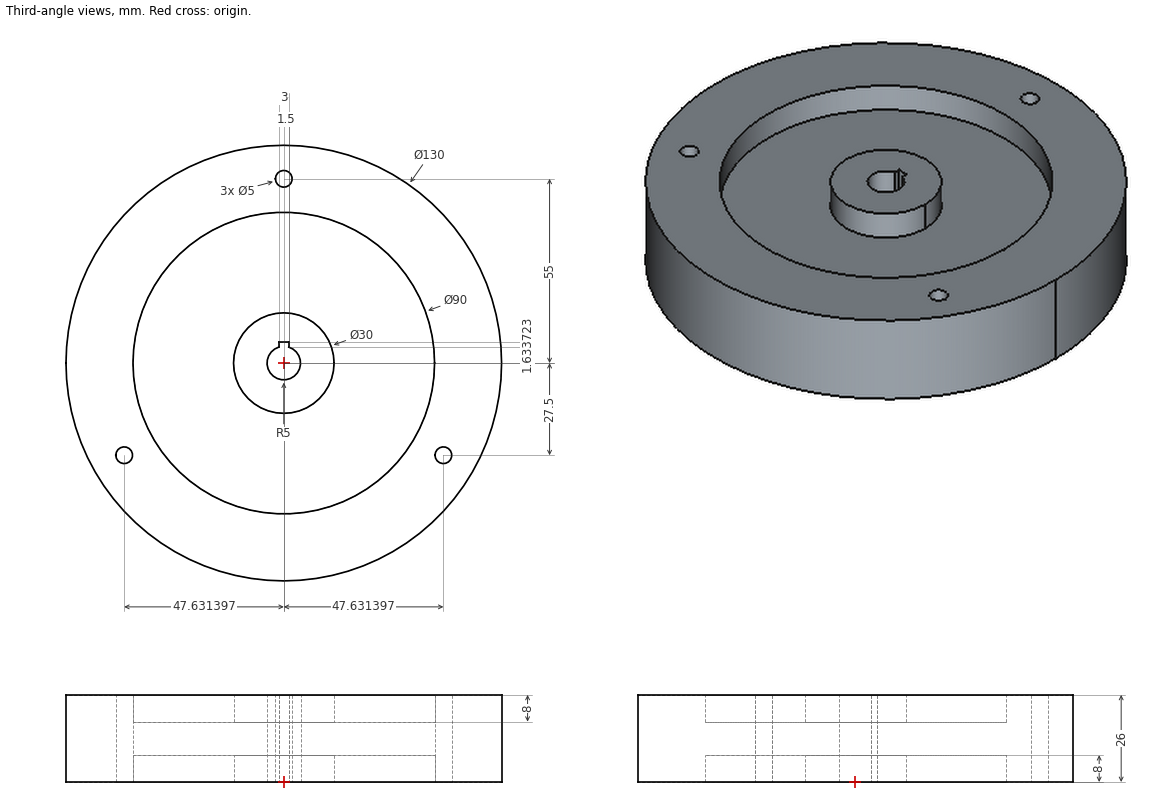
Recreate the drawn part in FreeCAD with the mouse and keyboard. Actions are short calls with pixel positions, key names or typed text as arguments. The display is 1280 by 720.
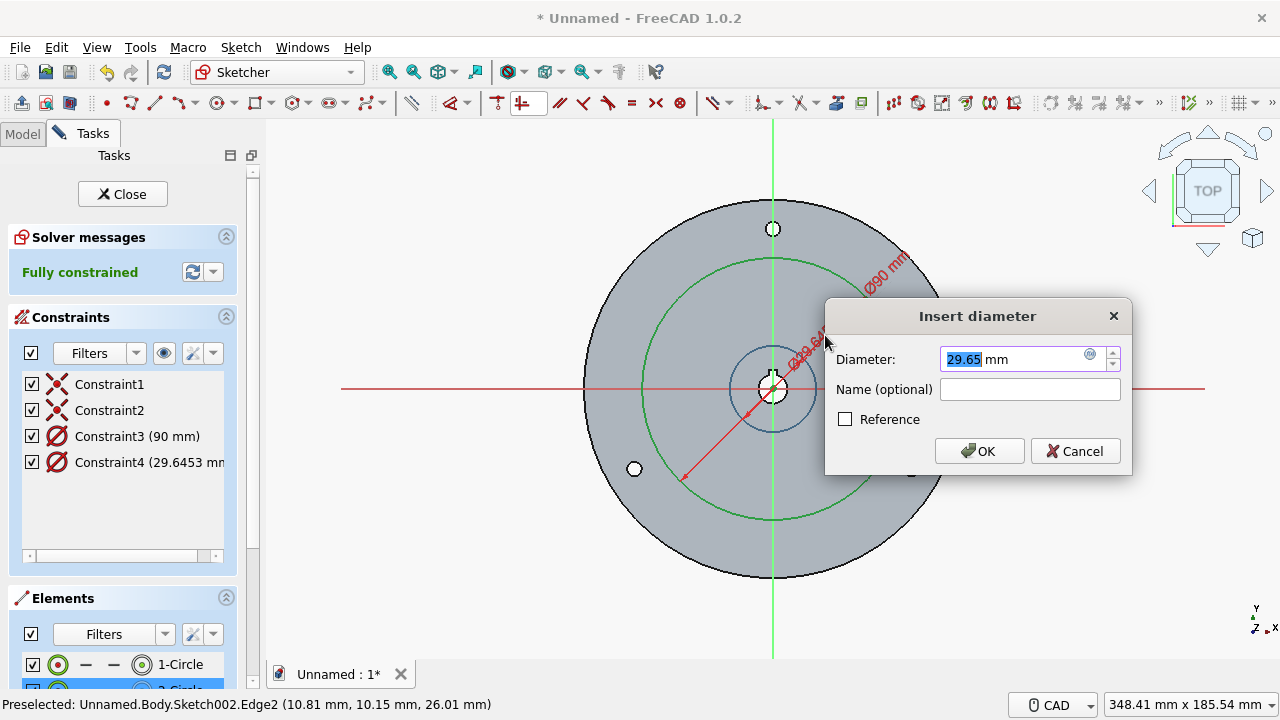
text(30)
key(Return)
key(Escape)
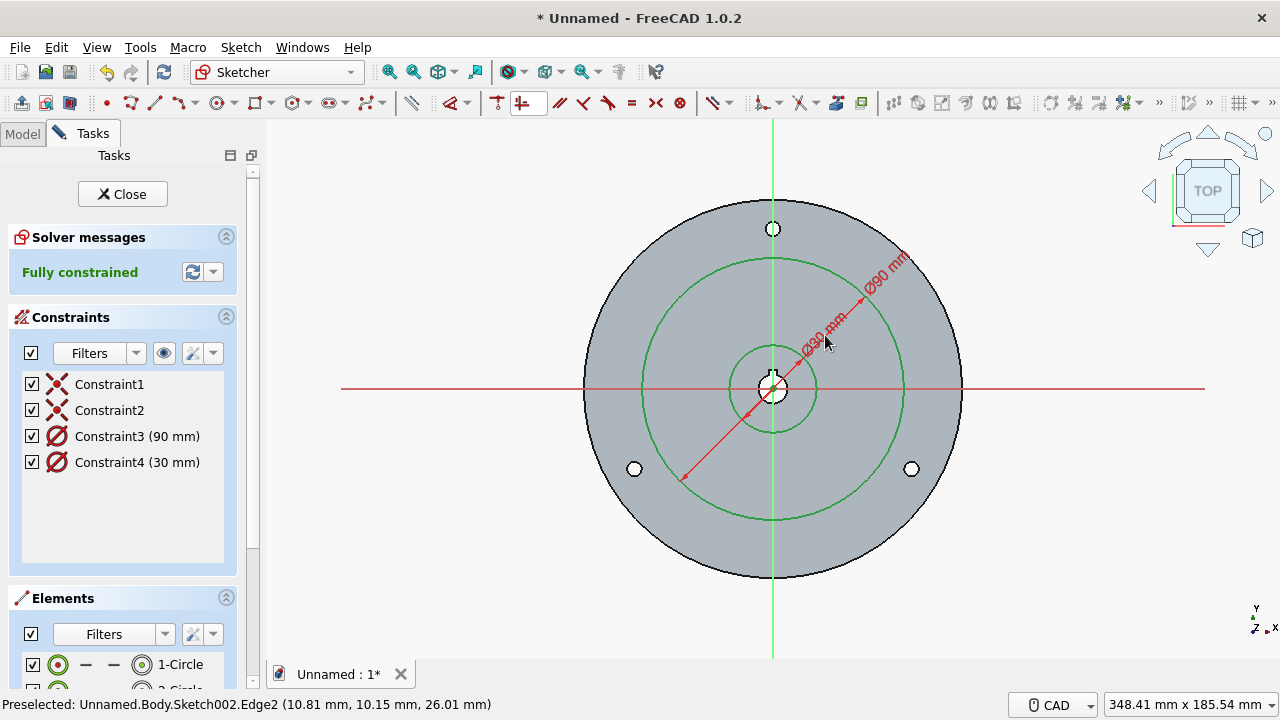
click(123, 194)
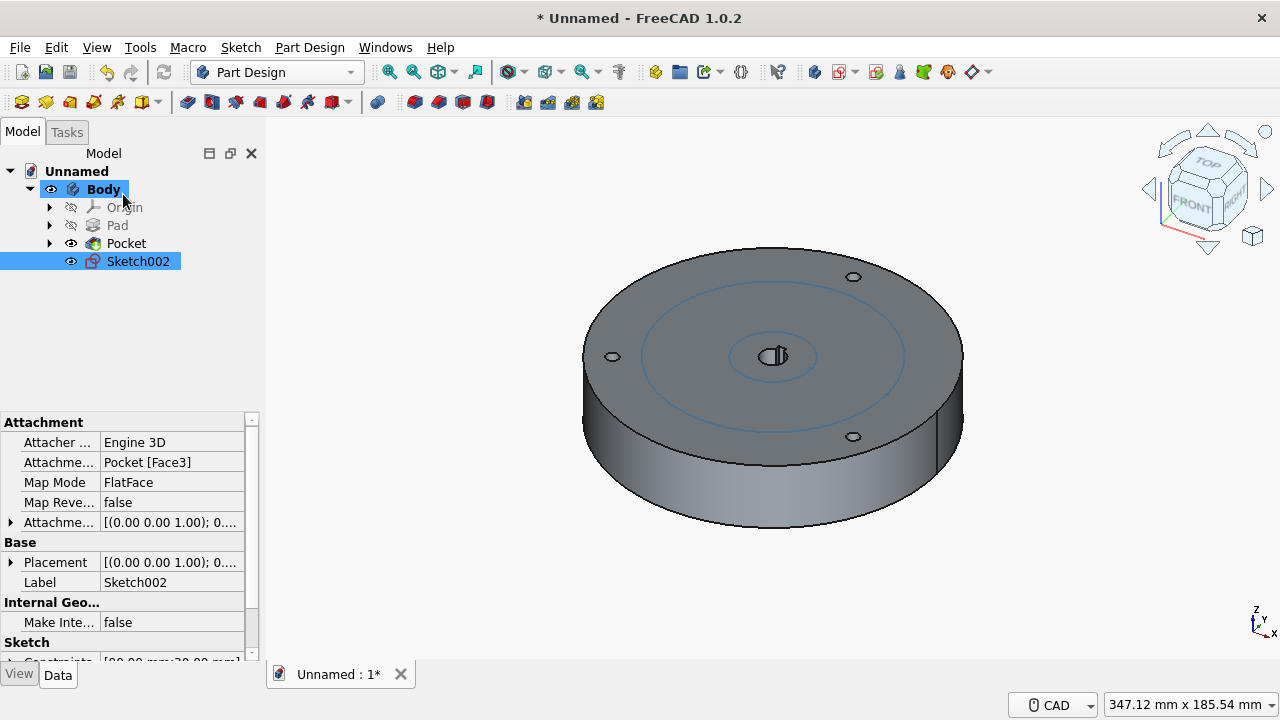
click(188, 102)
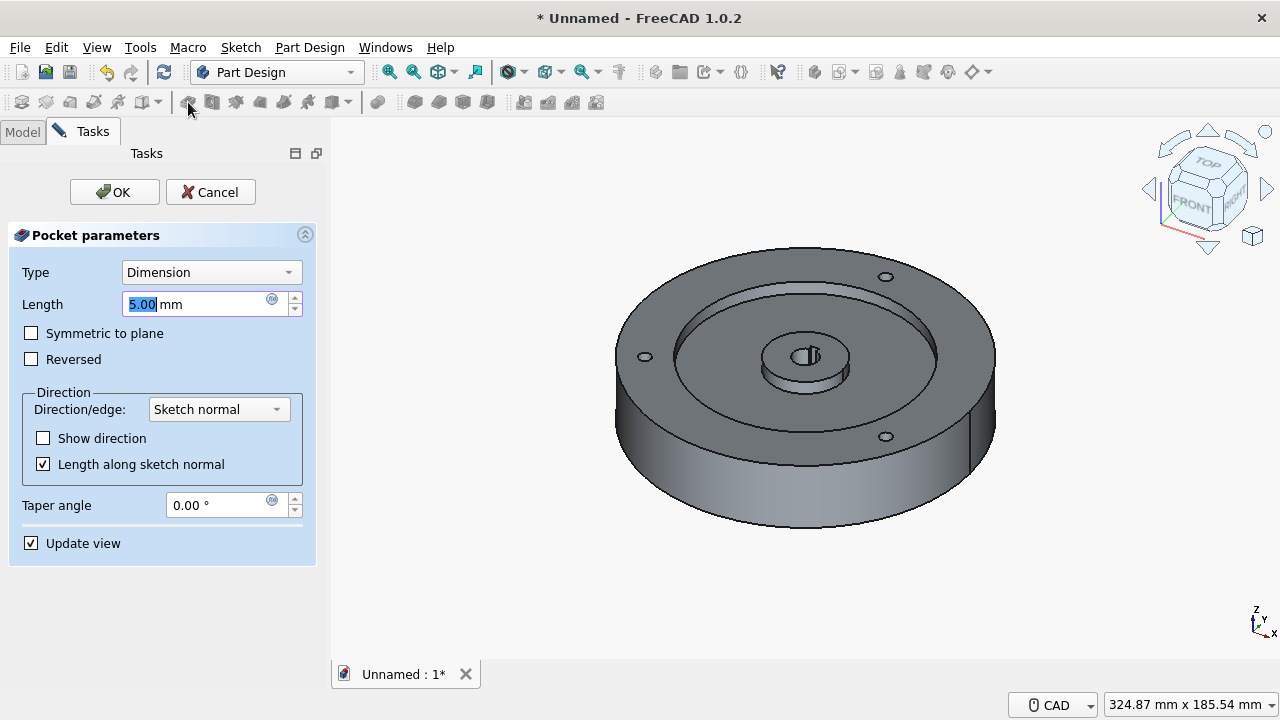
text(8)
key(Tab)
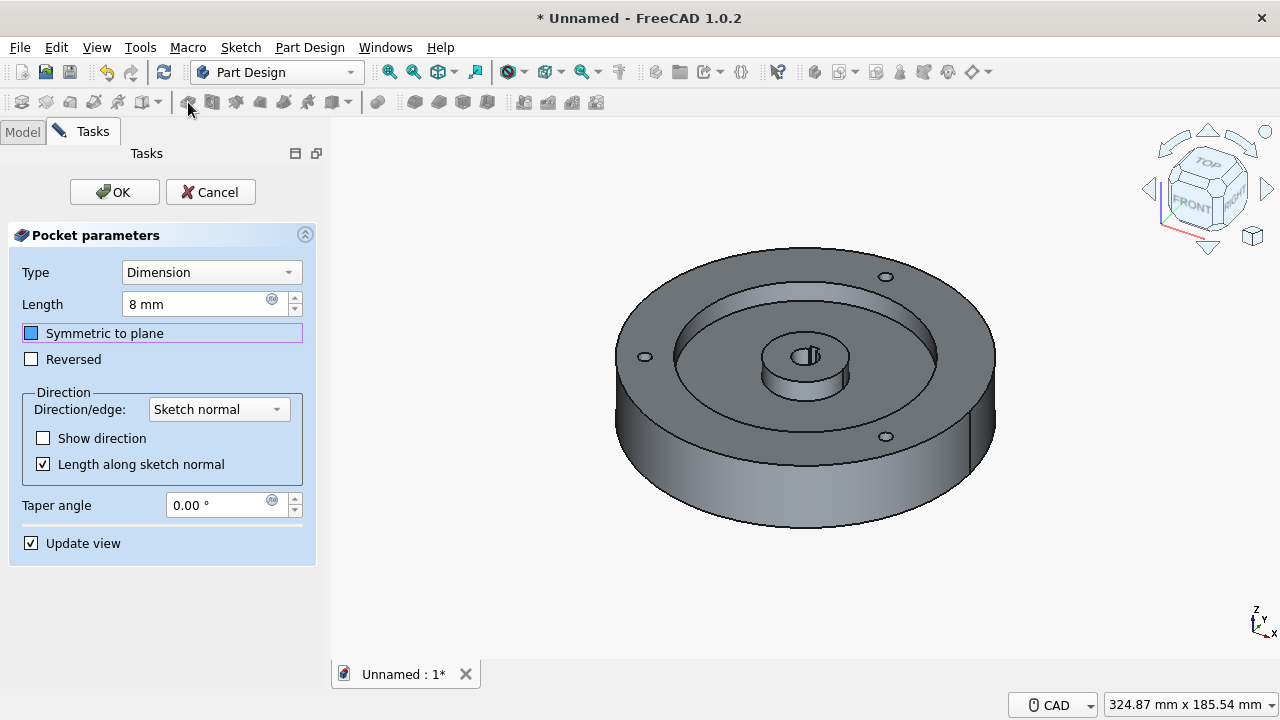
click(115, 192)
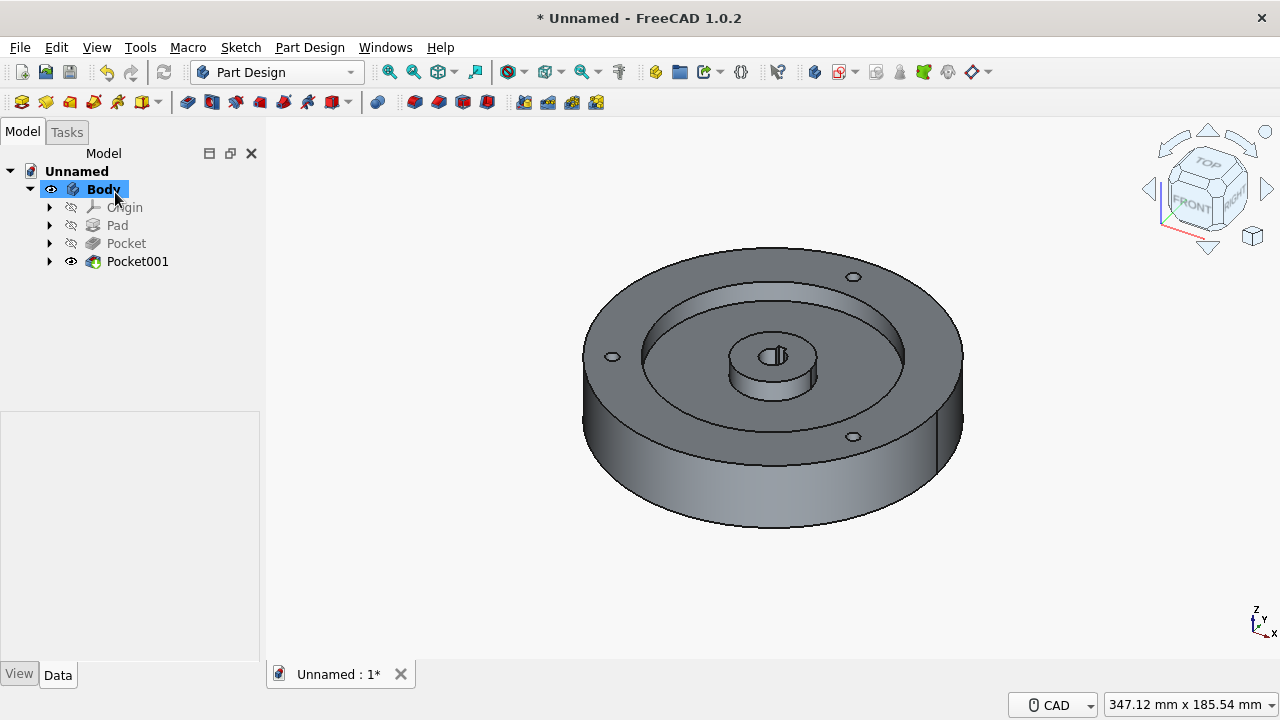
click(50, 207)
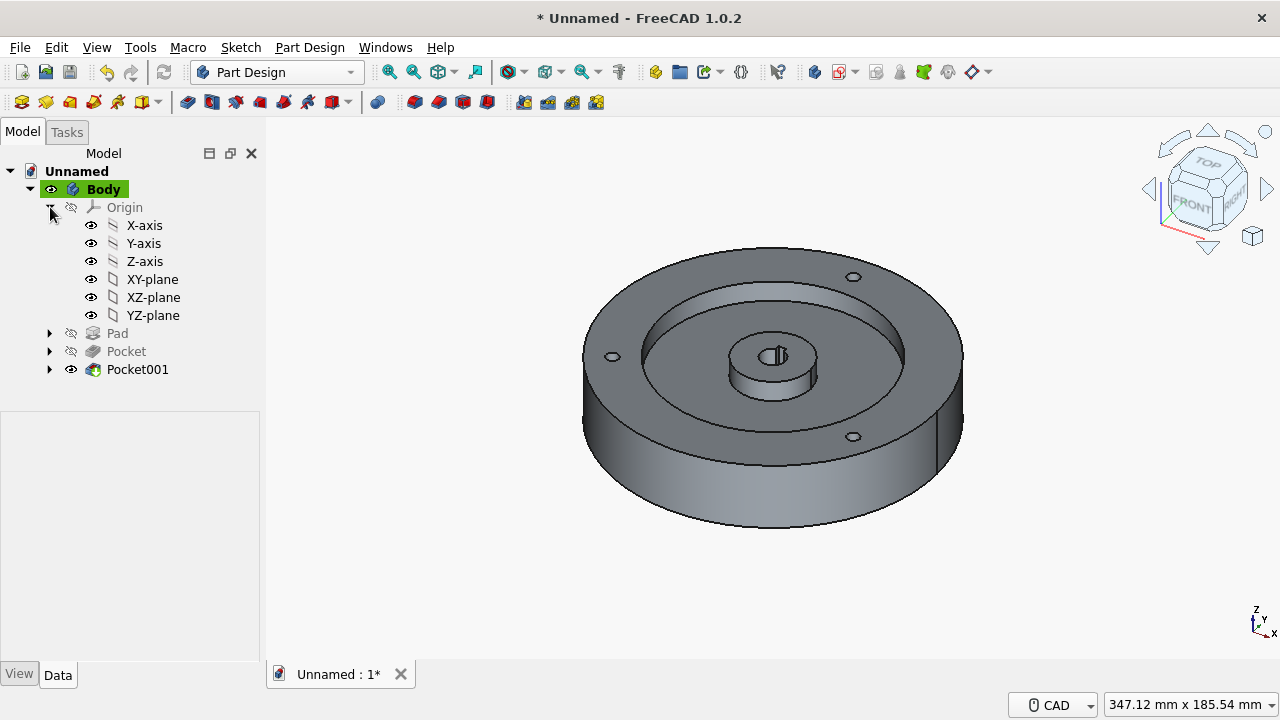
click(136, 279)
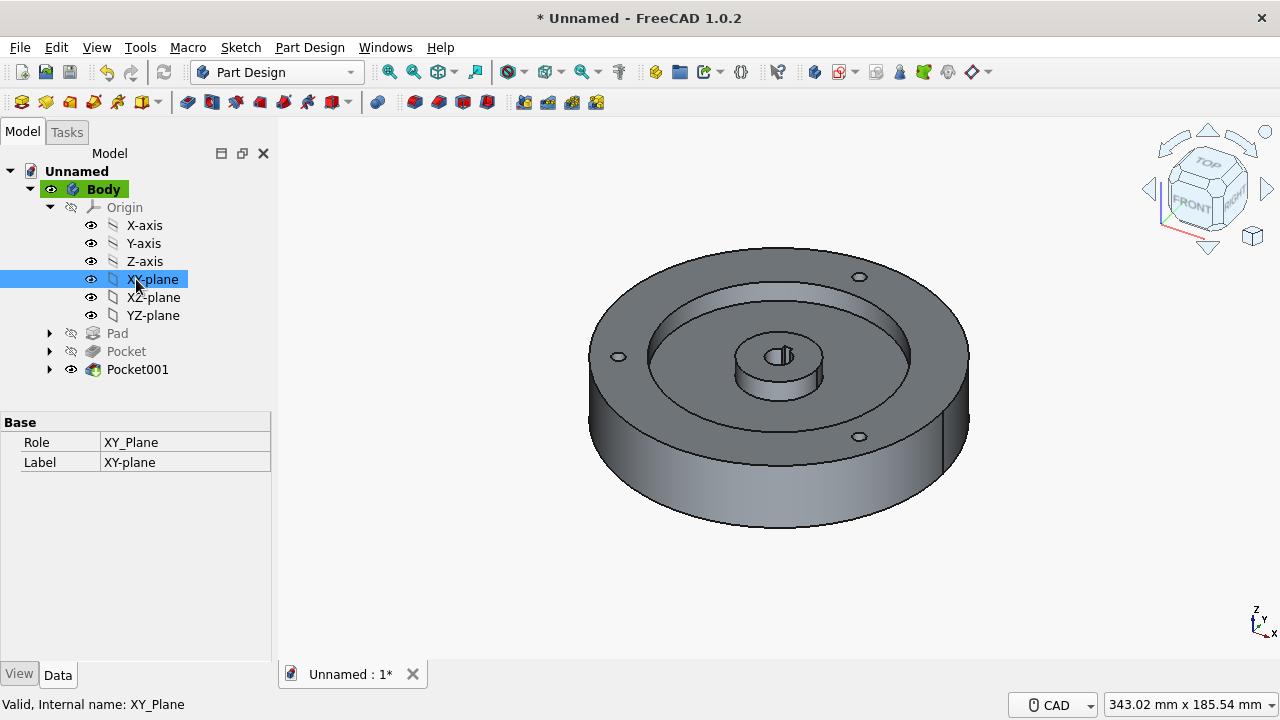
click(972, 72)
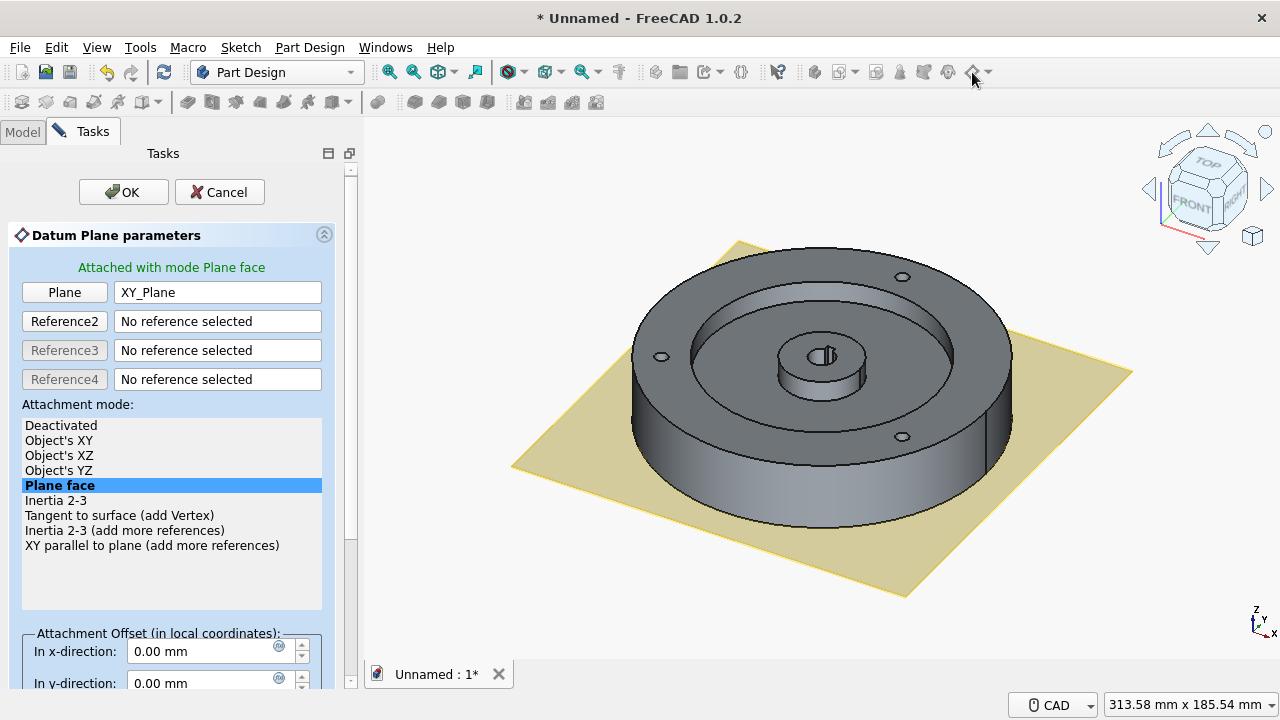
scroll(351, 426, down, 2)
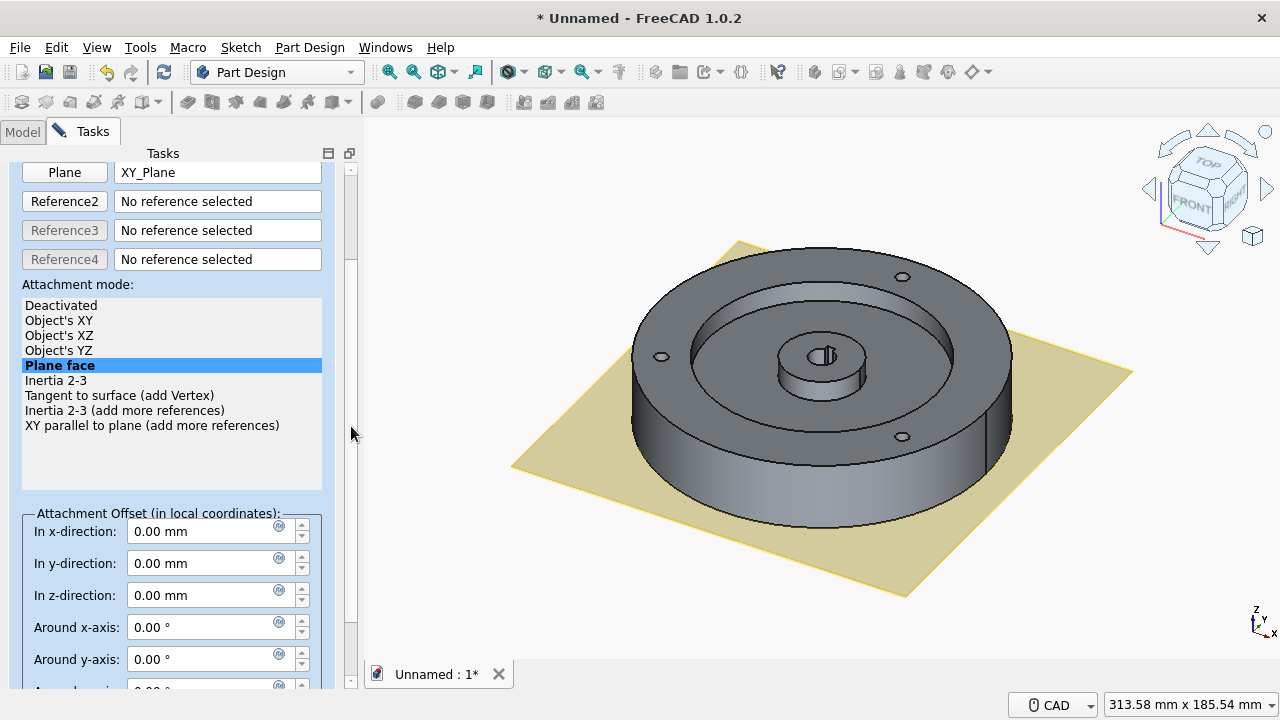
triple_click(210, 595)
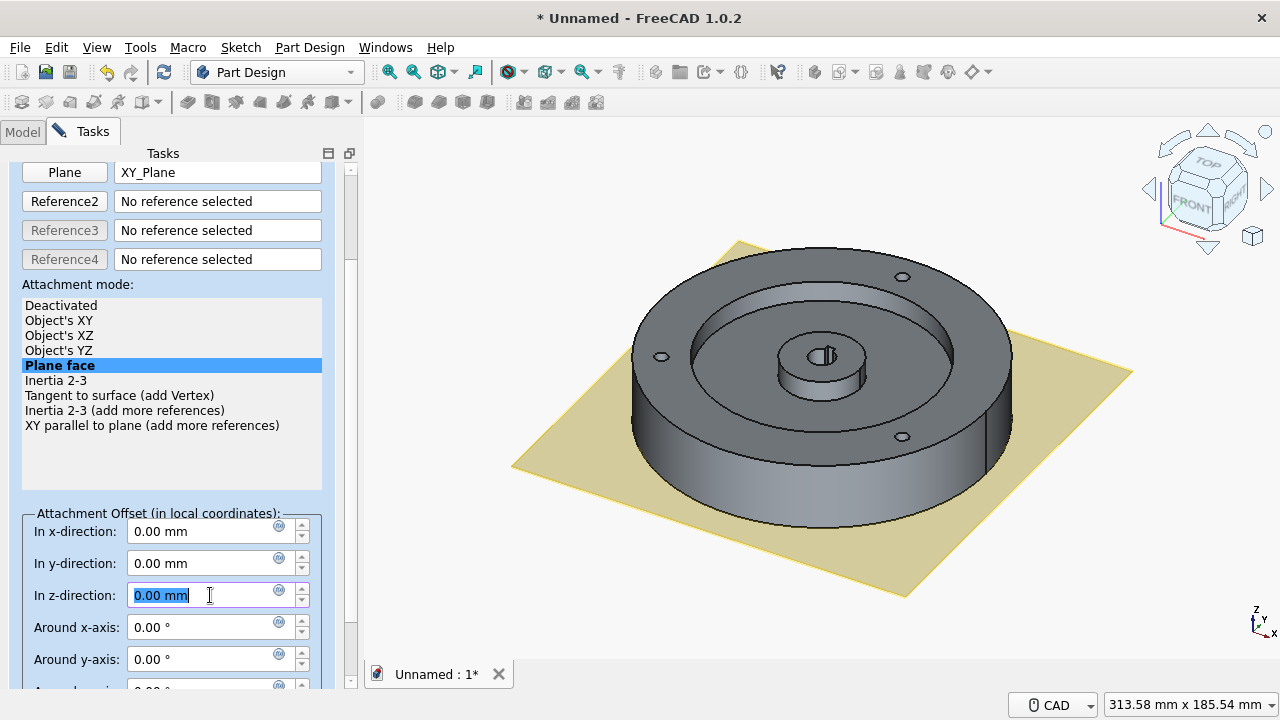
text(8)
key(Tab)